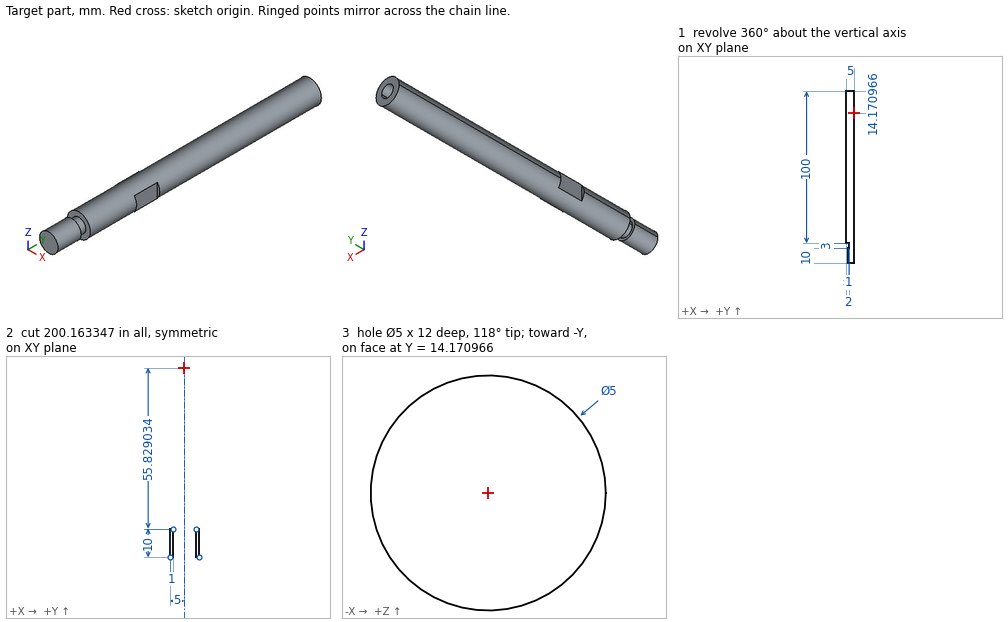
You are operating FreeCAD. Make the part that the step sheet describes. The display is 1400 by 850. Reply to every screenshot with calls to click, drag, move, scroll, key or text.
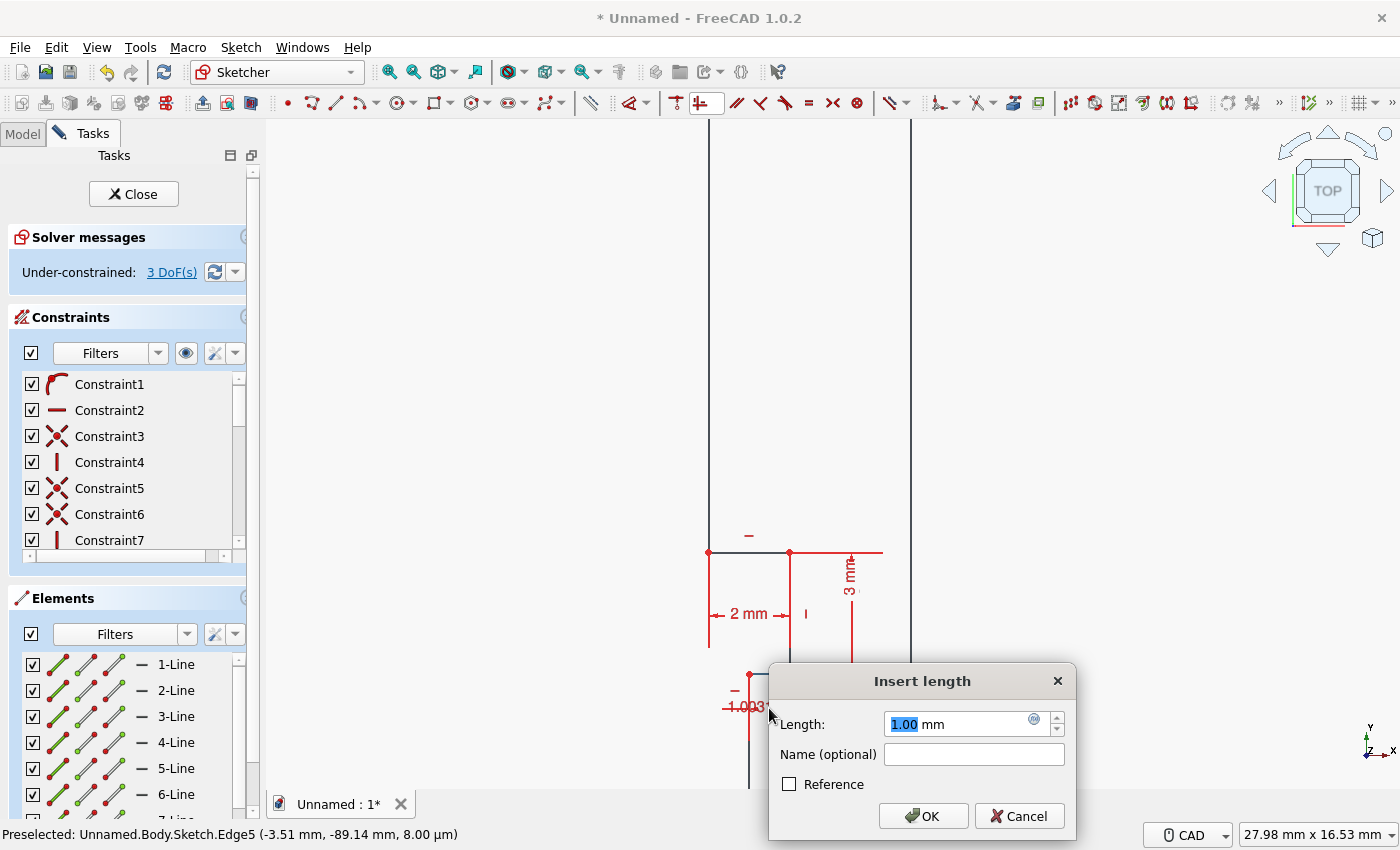
text(1)
key(Return)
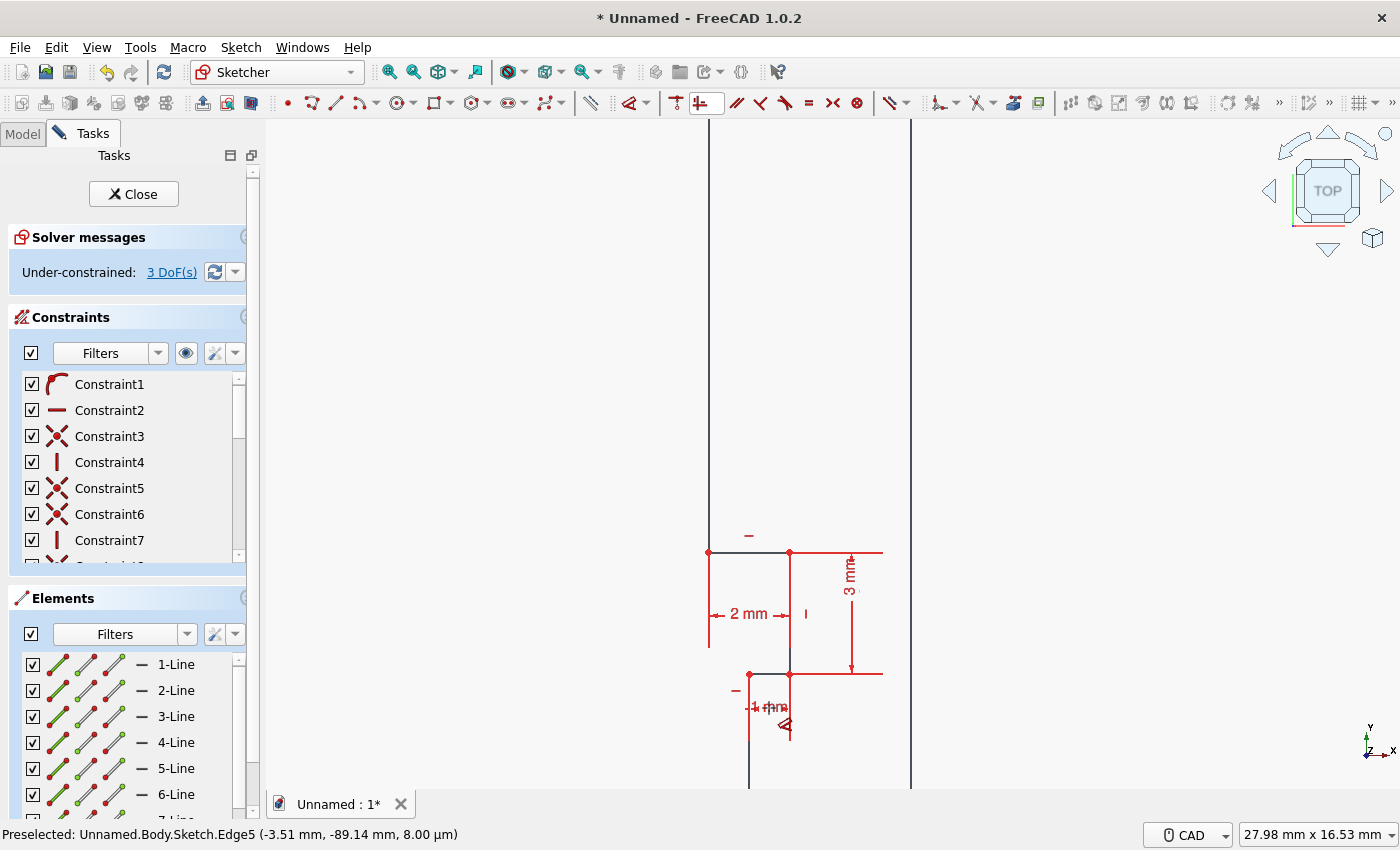
scroll(760, 621, down, 12)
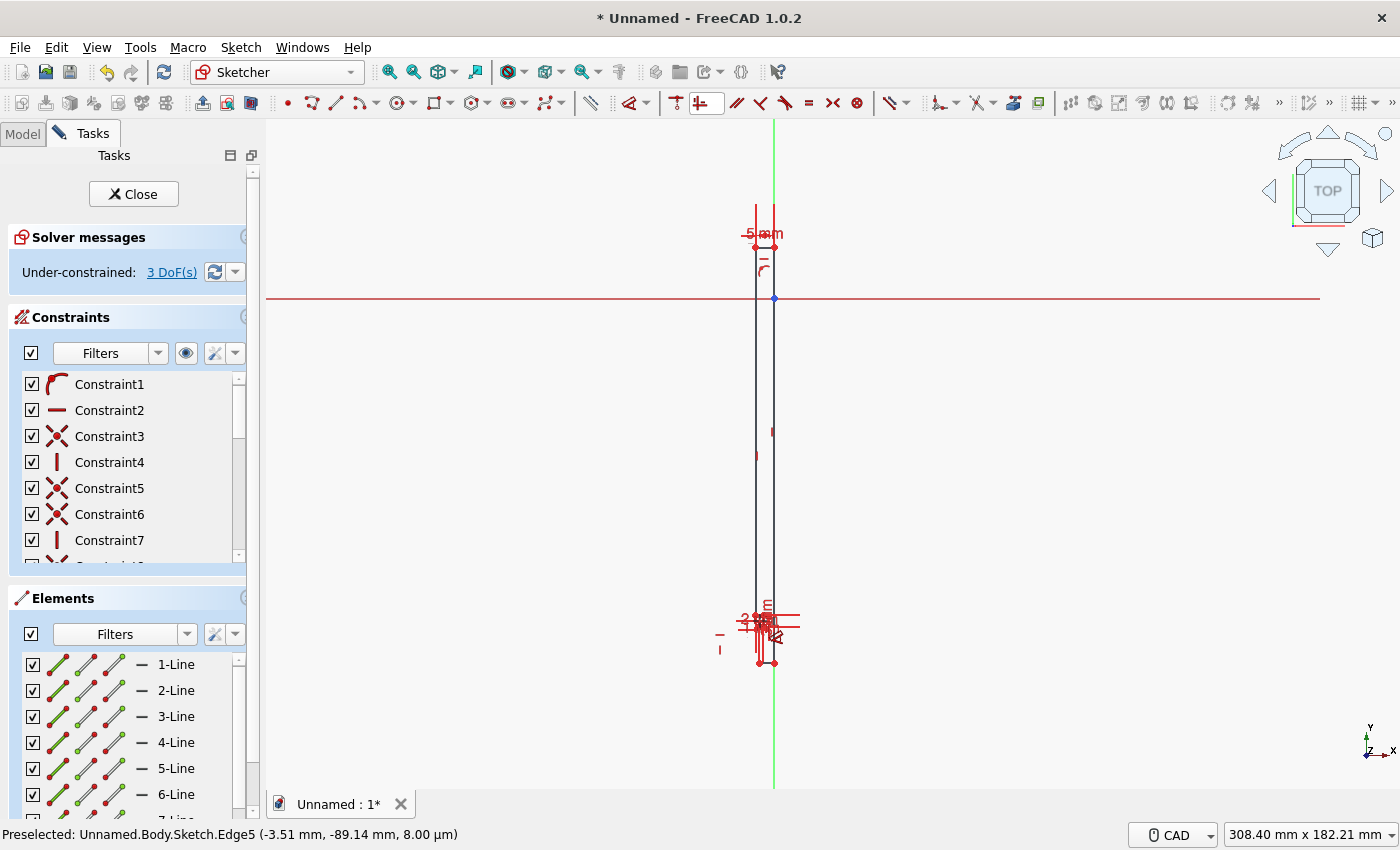
scroll(759, 634, up, 4)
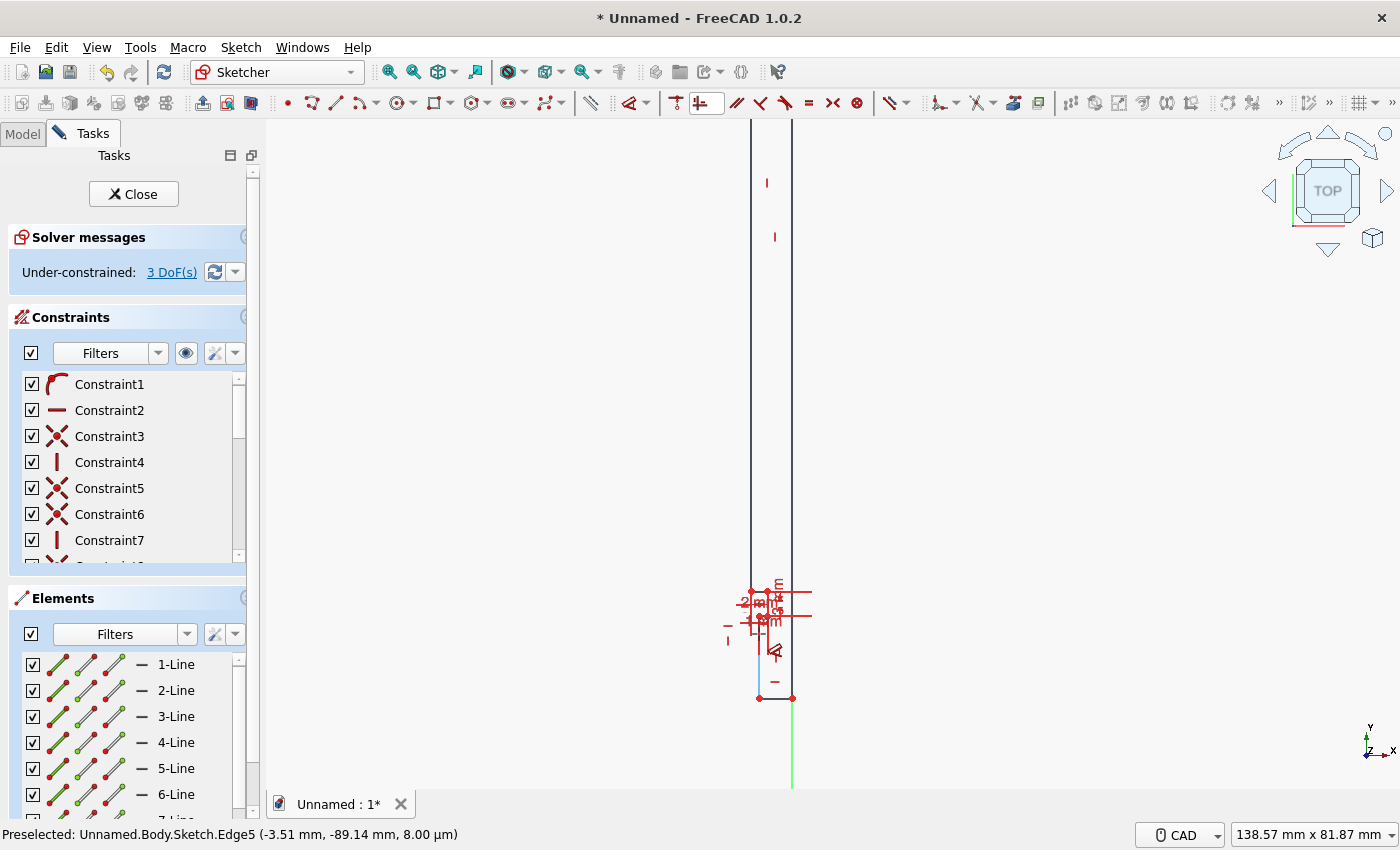
click(759, 633)
click(725, 658)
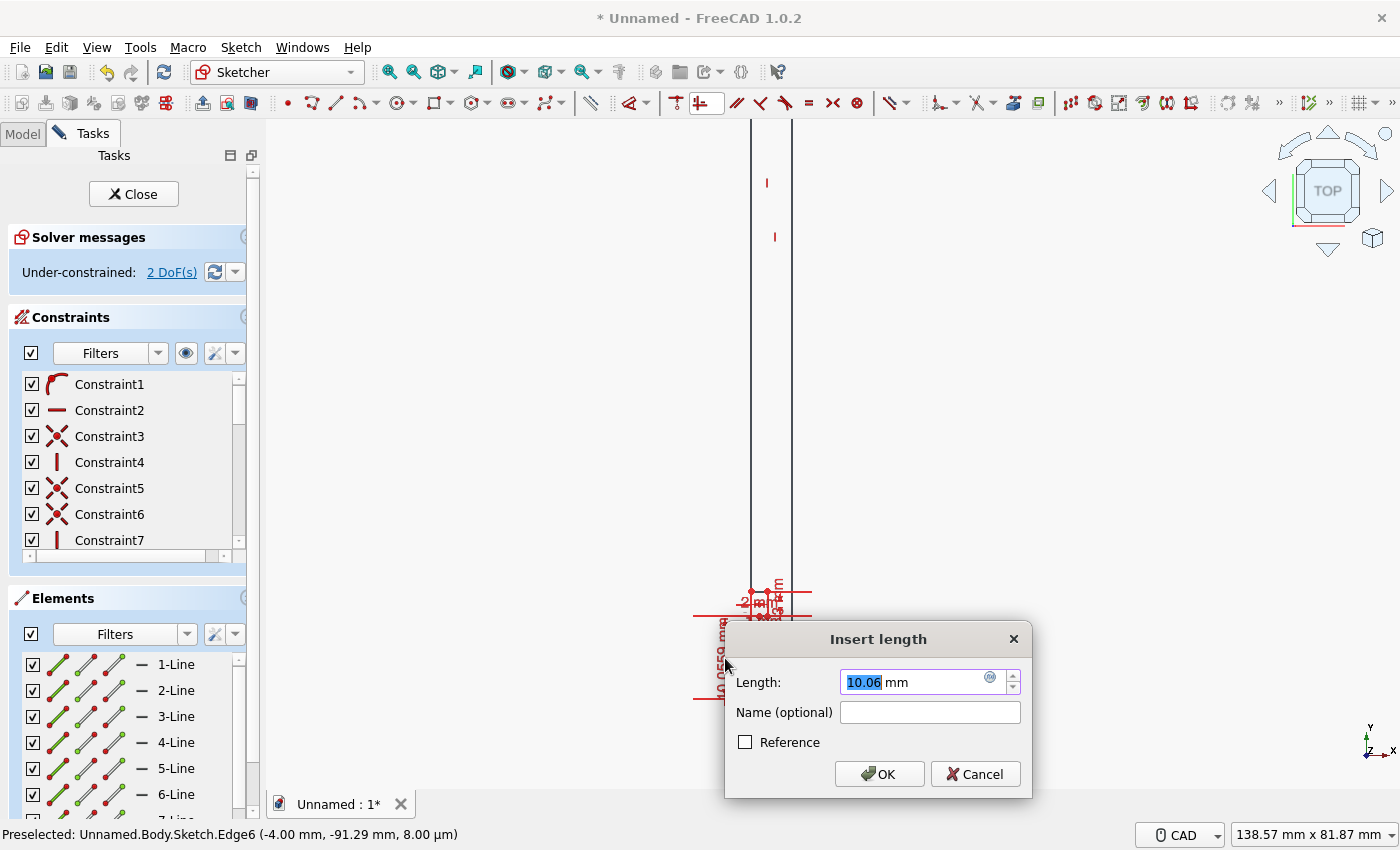
text(10)
key(Return)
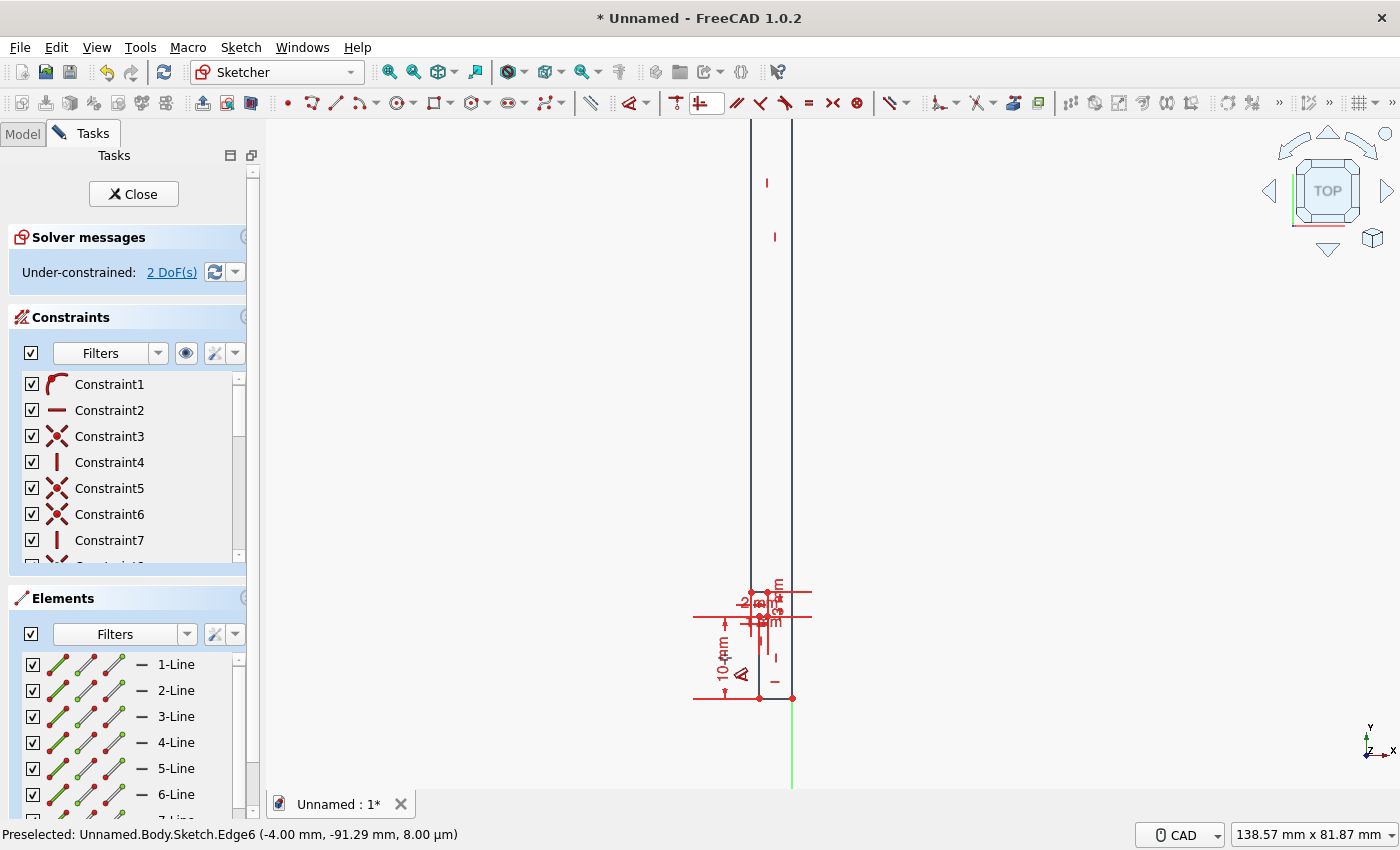
click(751, 347)
click(717, 370)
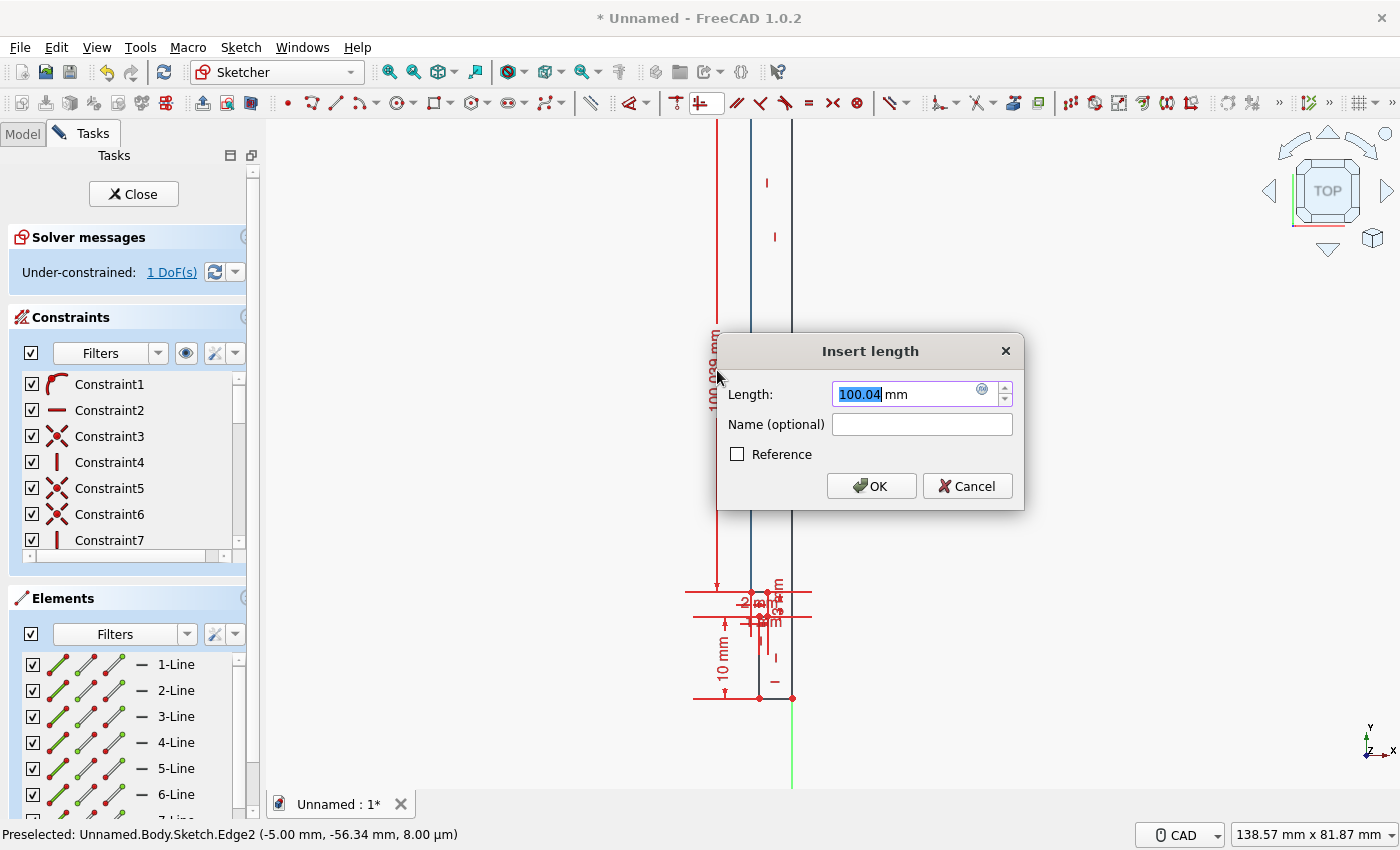
text(100)
key(Return)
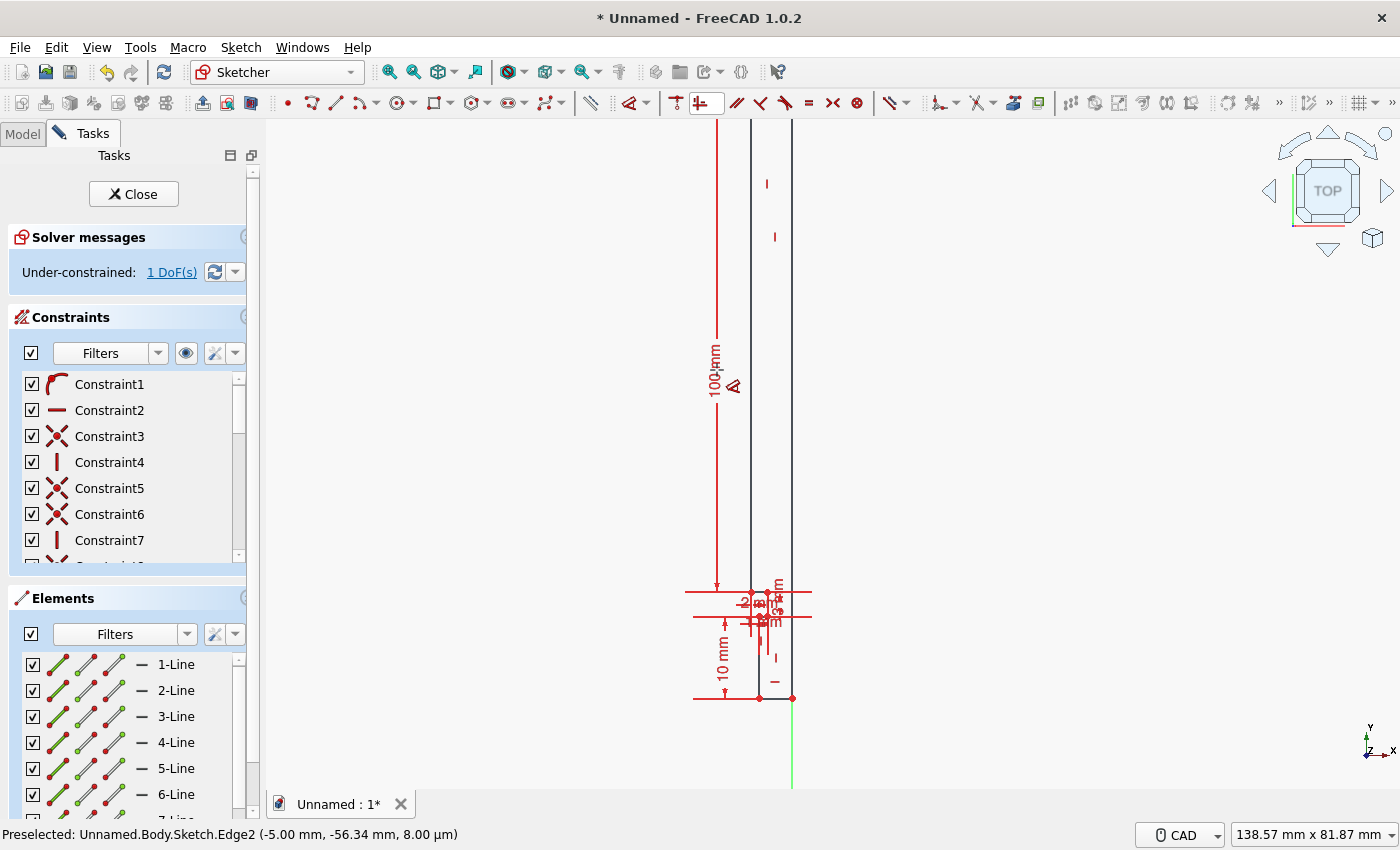
scroll(759, 634, down, 4)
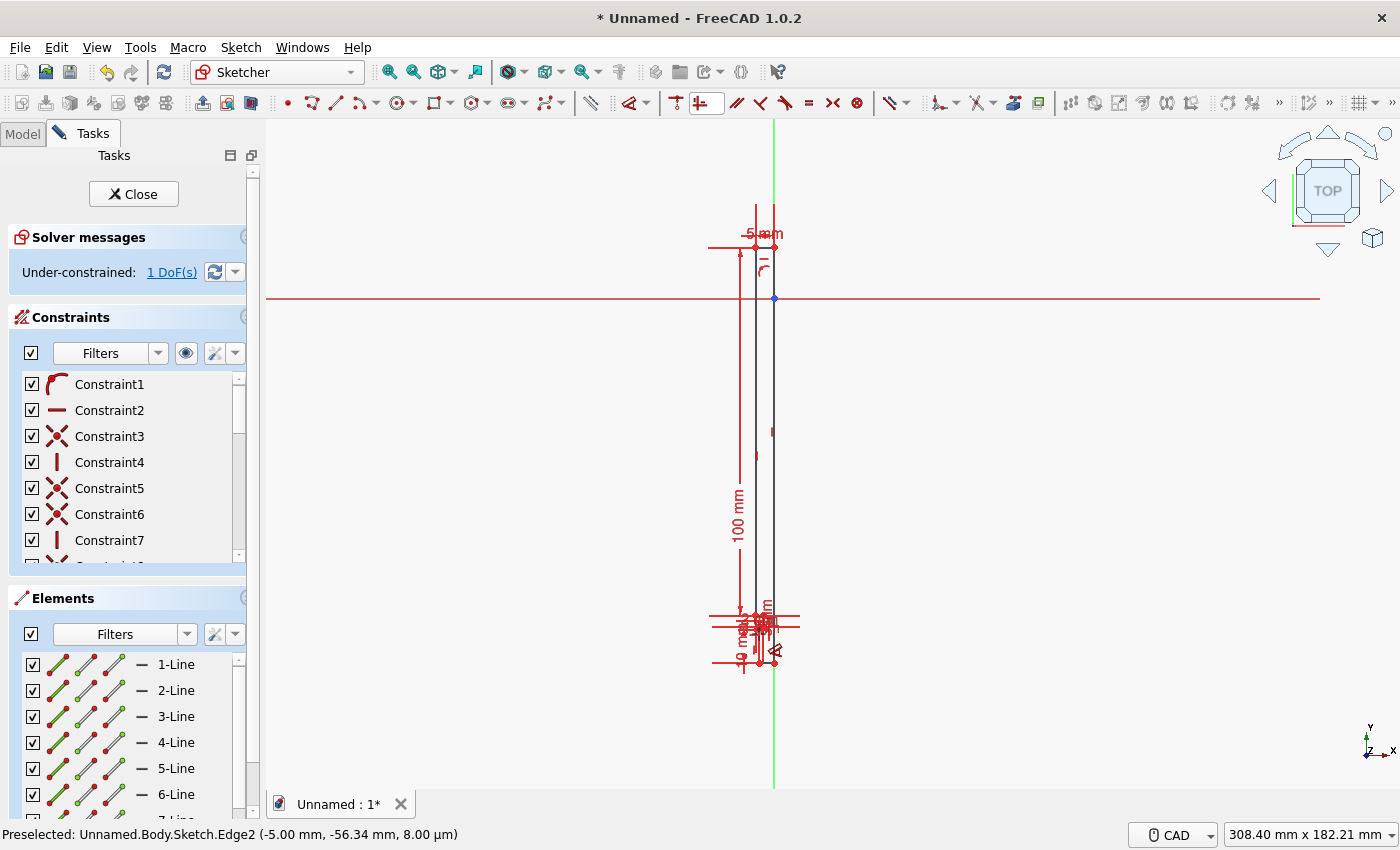
click(774, 248)
click(808, 273)